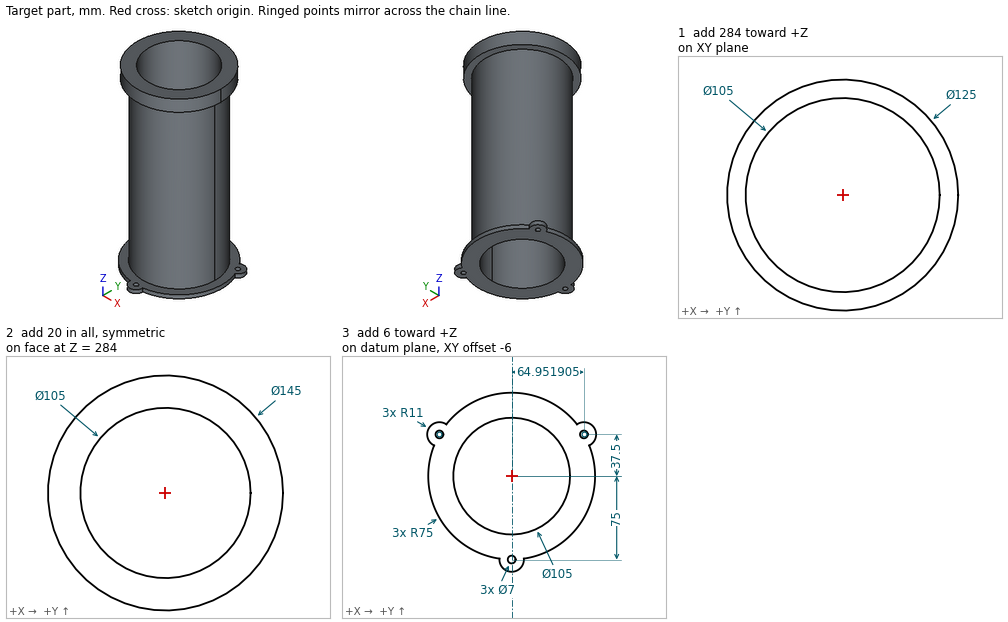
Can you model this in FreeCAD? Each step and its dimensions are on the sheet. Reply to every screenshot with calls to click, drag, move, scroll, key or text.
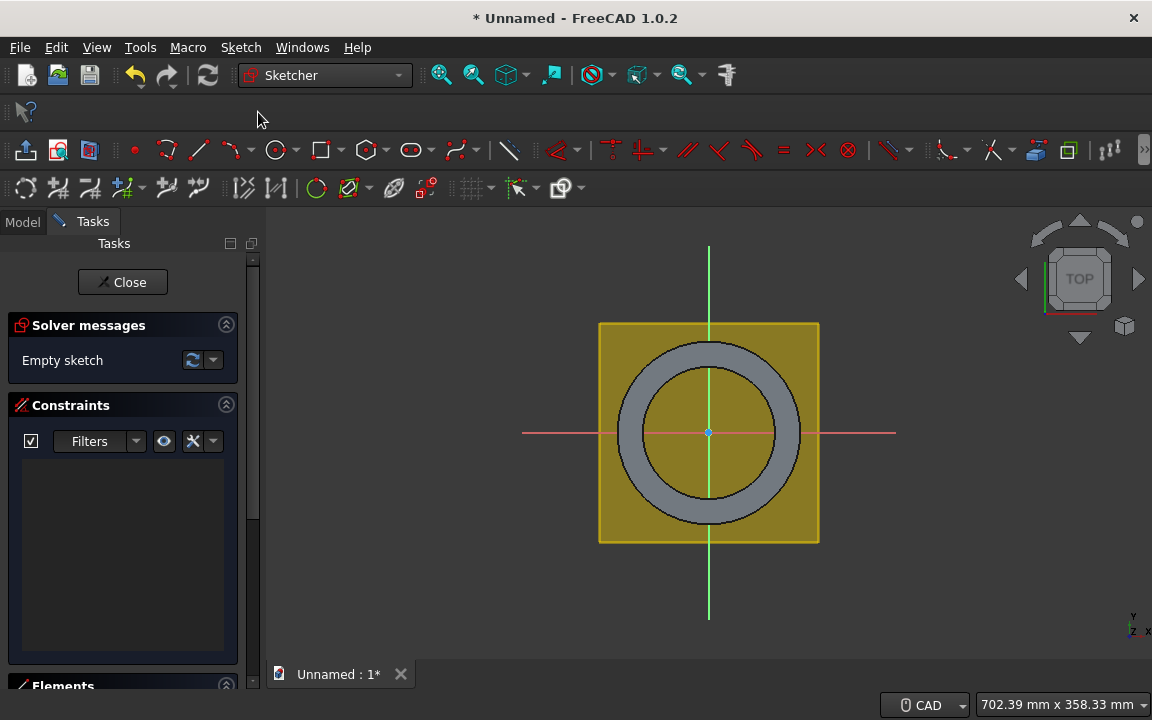
click(90, 150)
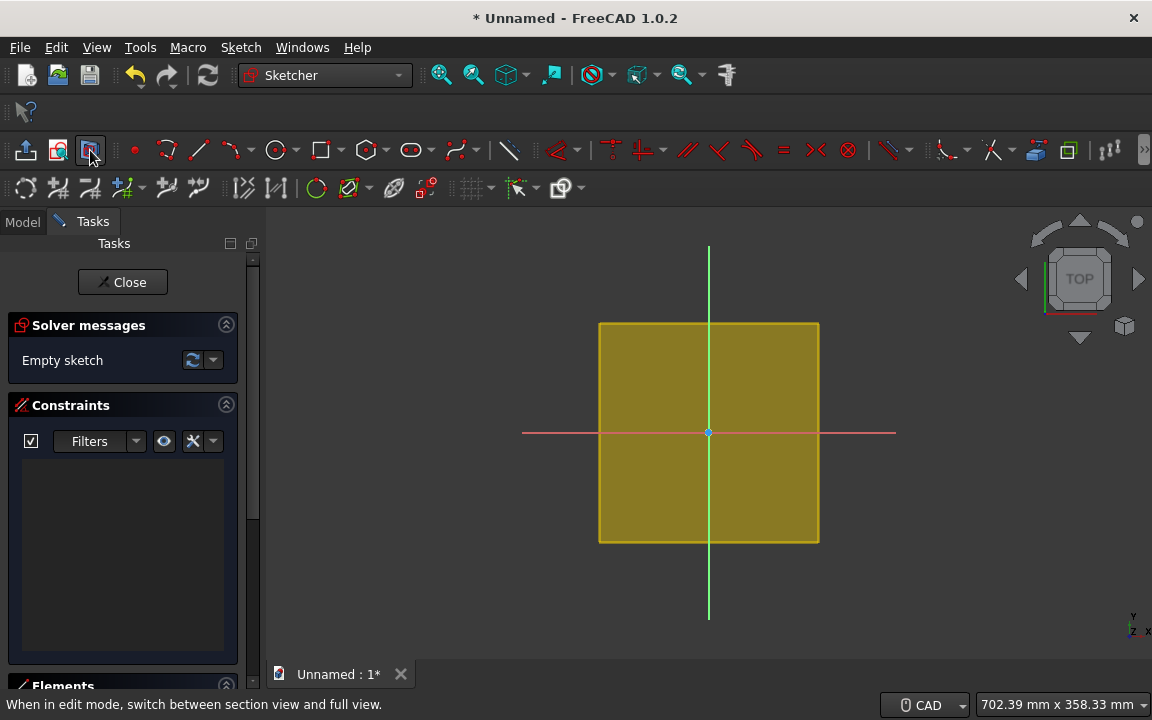
scroll(848, 454, up, 2)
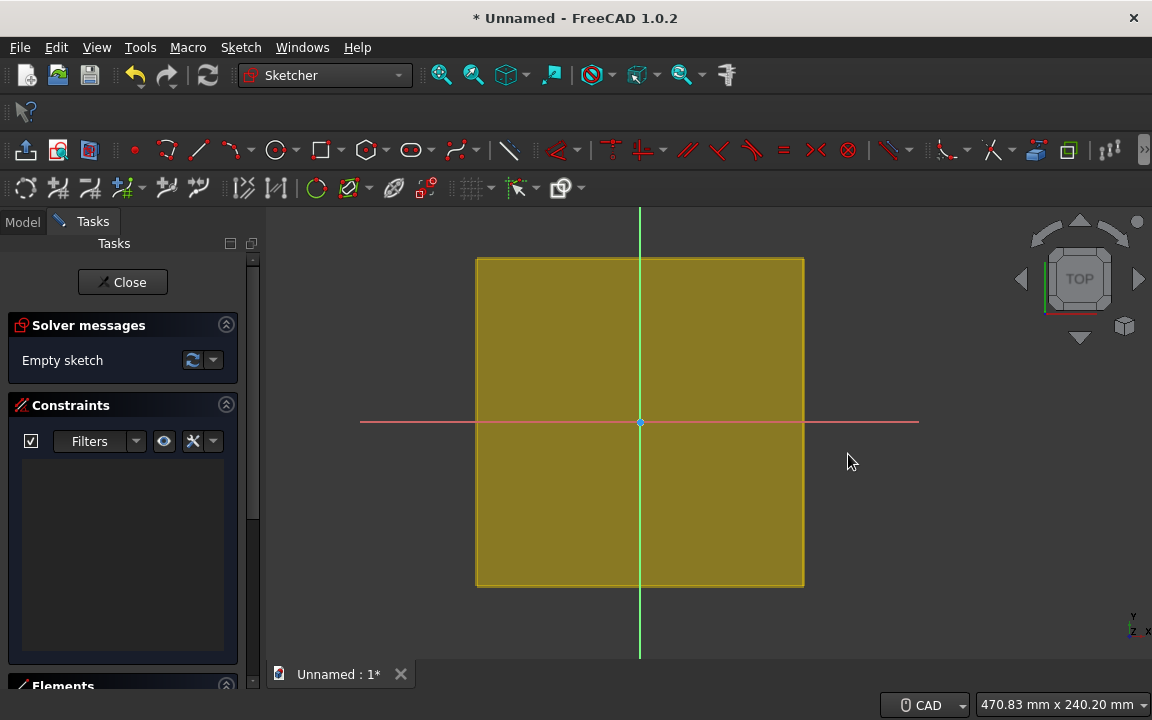
click(232, 150)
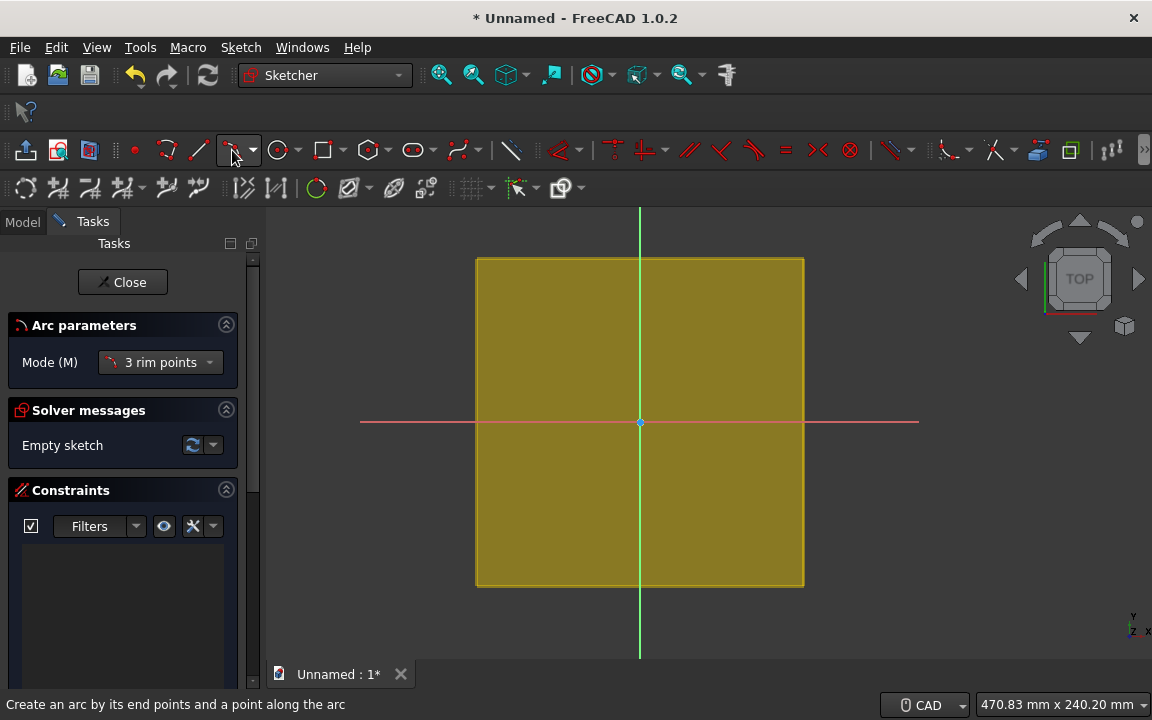
click(530, 335)
click(751, 335)
click(665, 284)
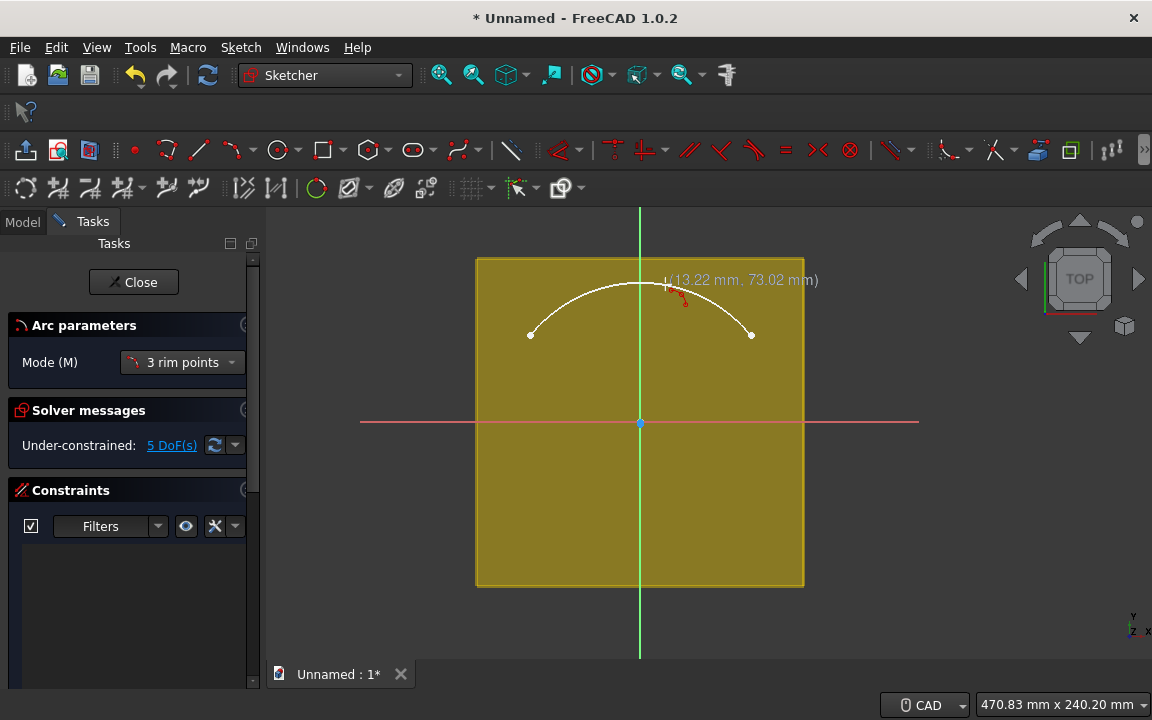
click(751, 336)
click(771, 370)
click(780, 341)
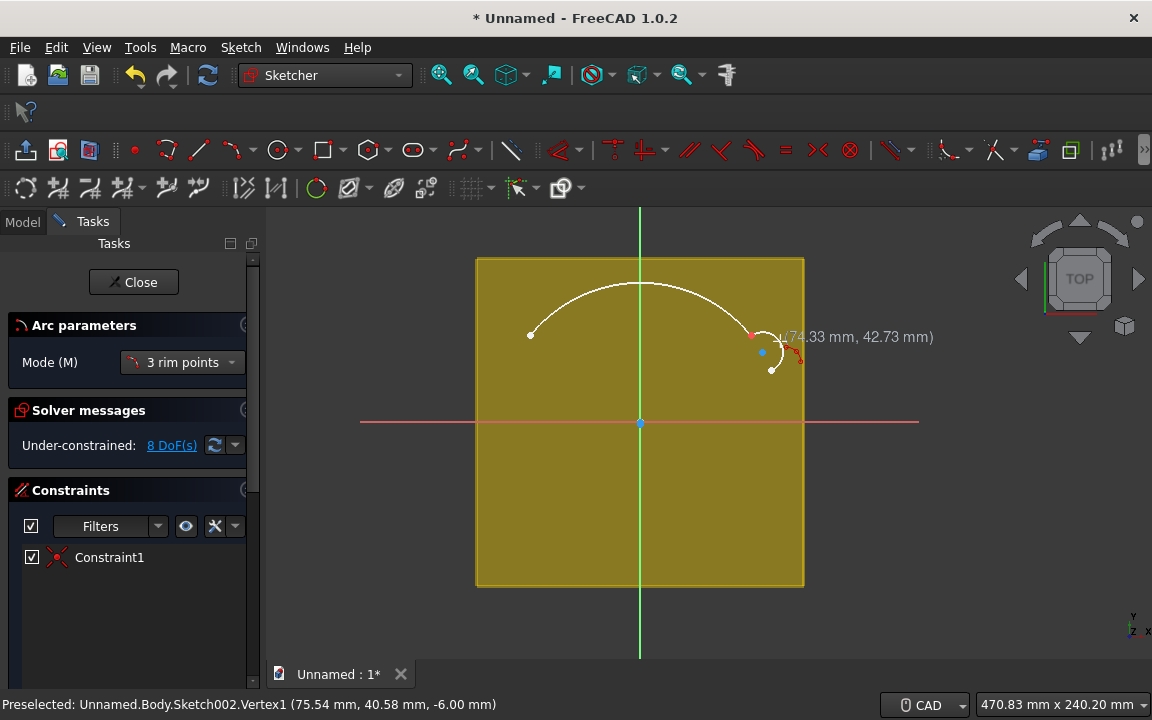
click(771, 371)
click(661, 562)
click(762, 493)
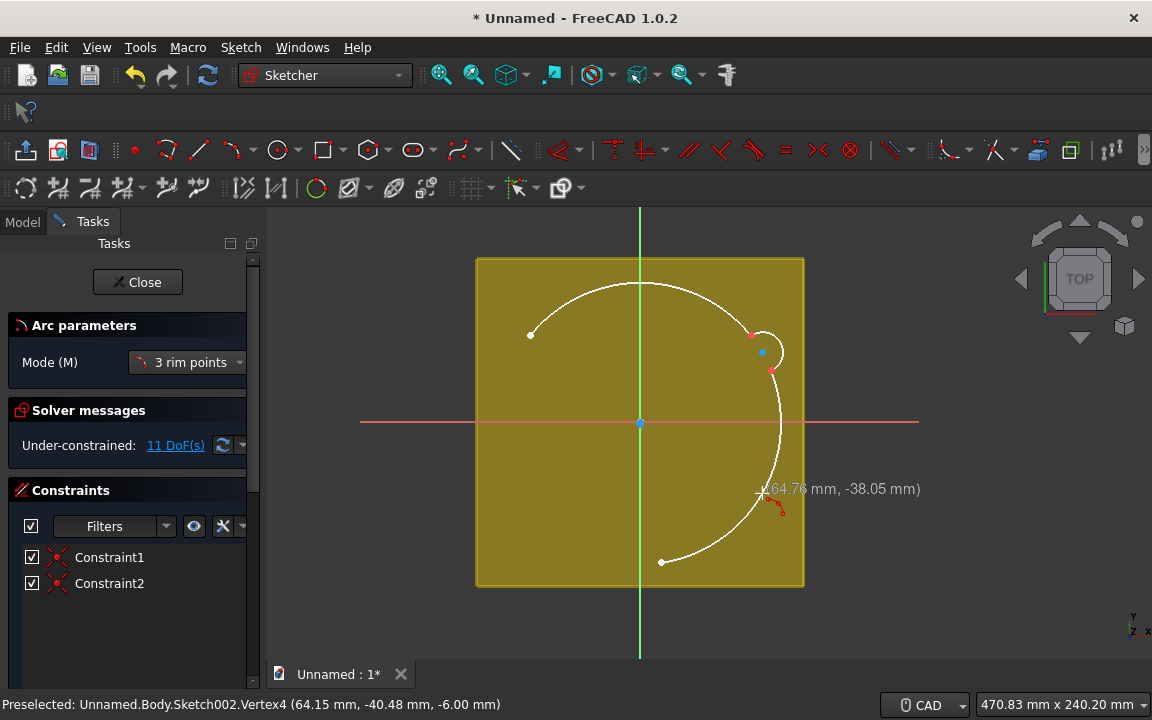
click(661, 563)
click(619, 562)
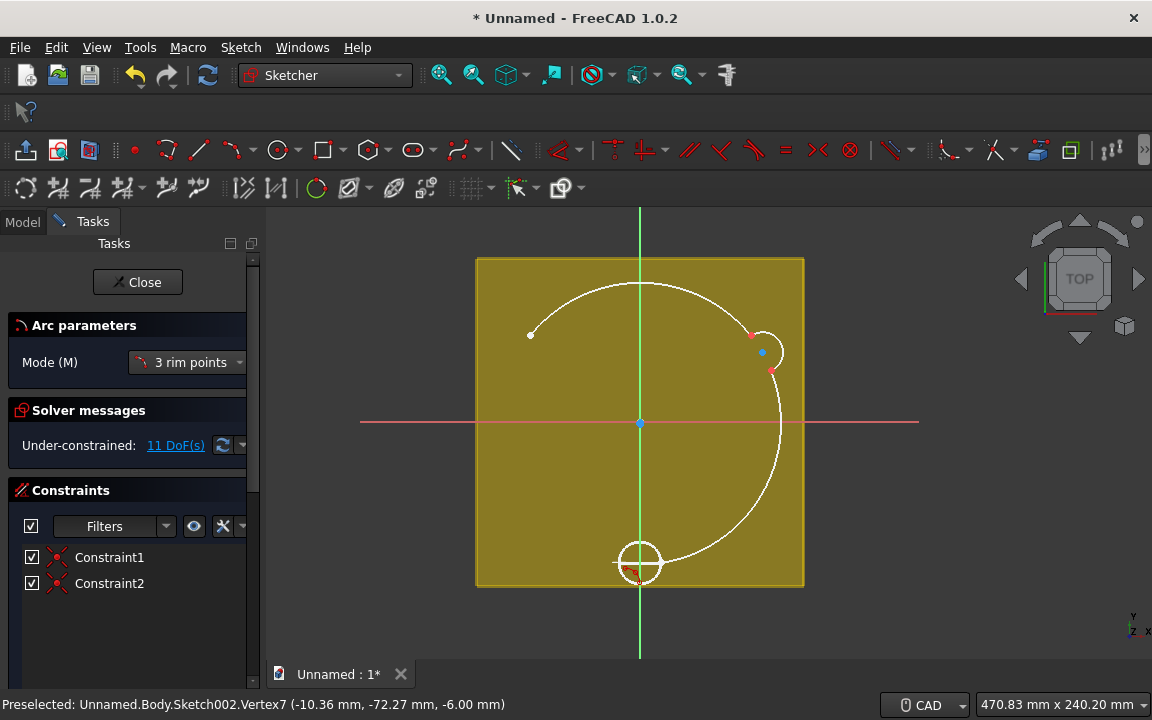
scroll(653, 580, up, 2)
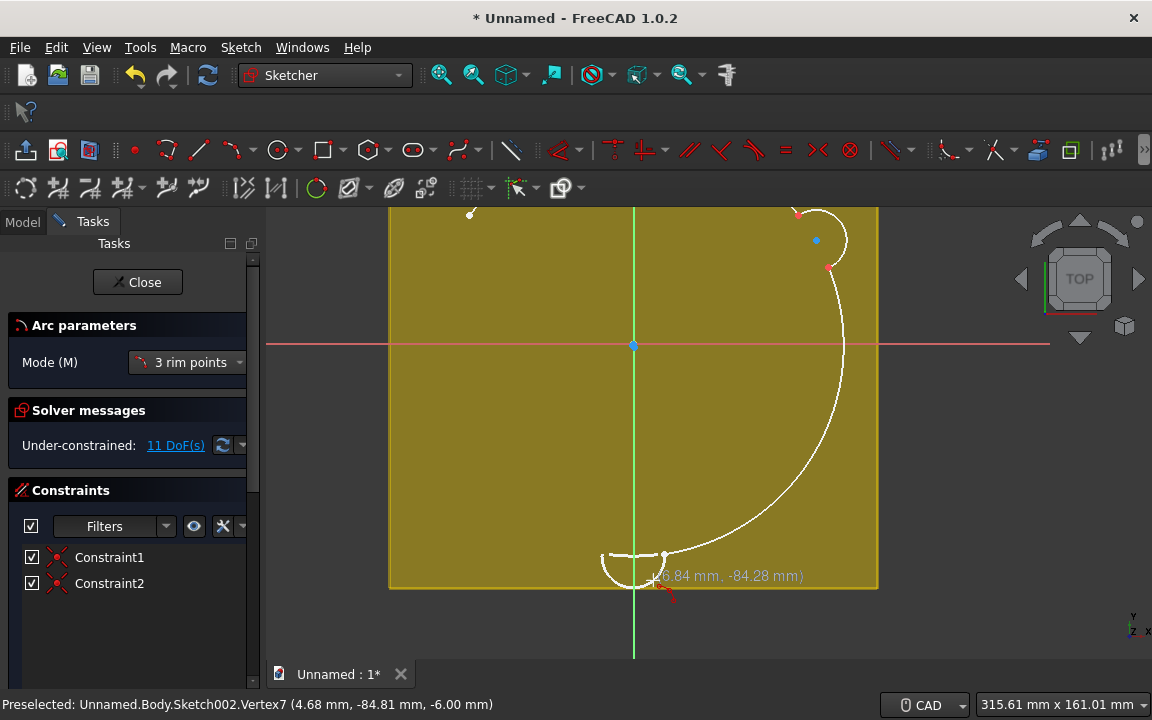
click(652, 579)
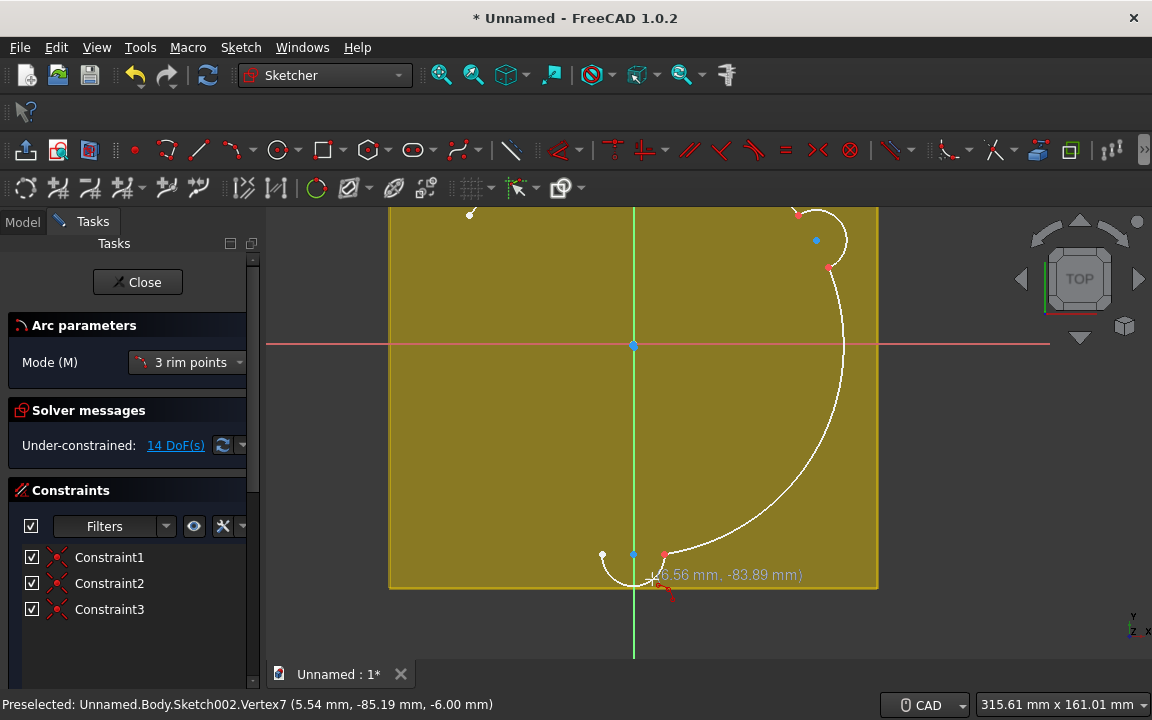
click(602, 554)
click(438, 267)
click(451, 450)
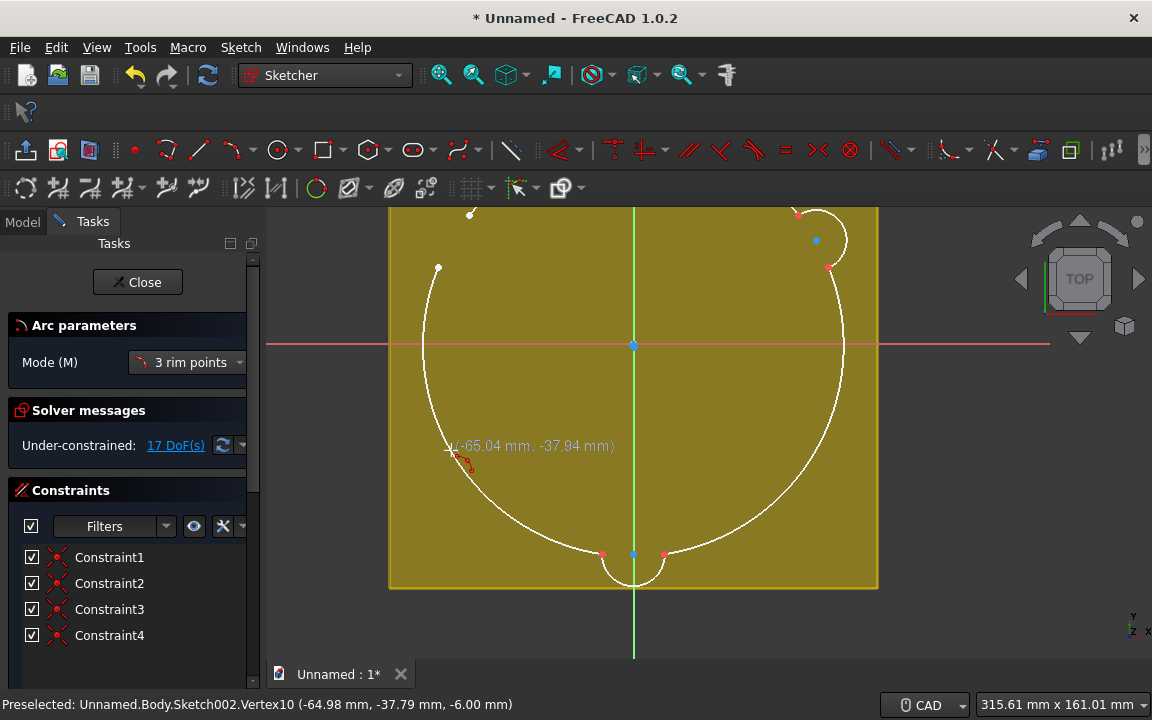
click(438, 268)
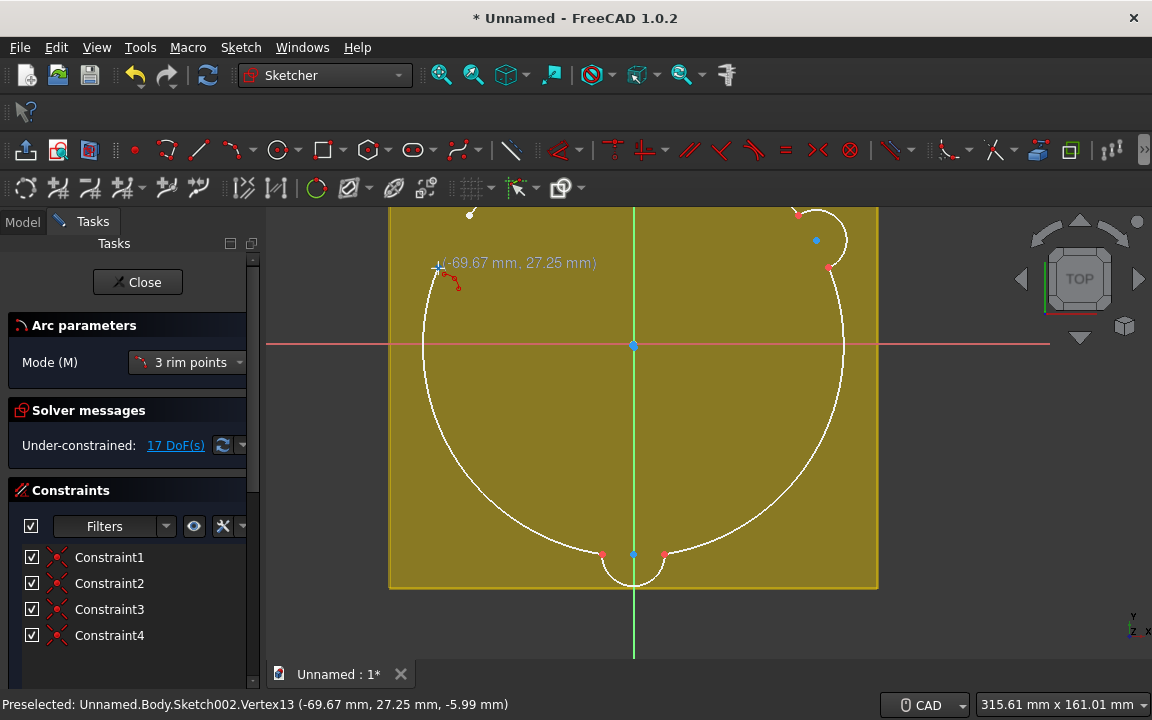
scroll(655, 582, down, 2)